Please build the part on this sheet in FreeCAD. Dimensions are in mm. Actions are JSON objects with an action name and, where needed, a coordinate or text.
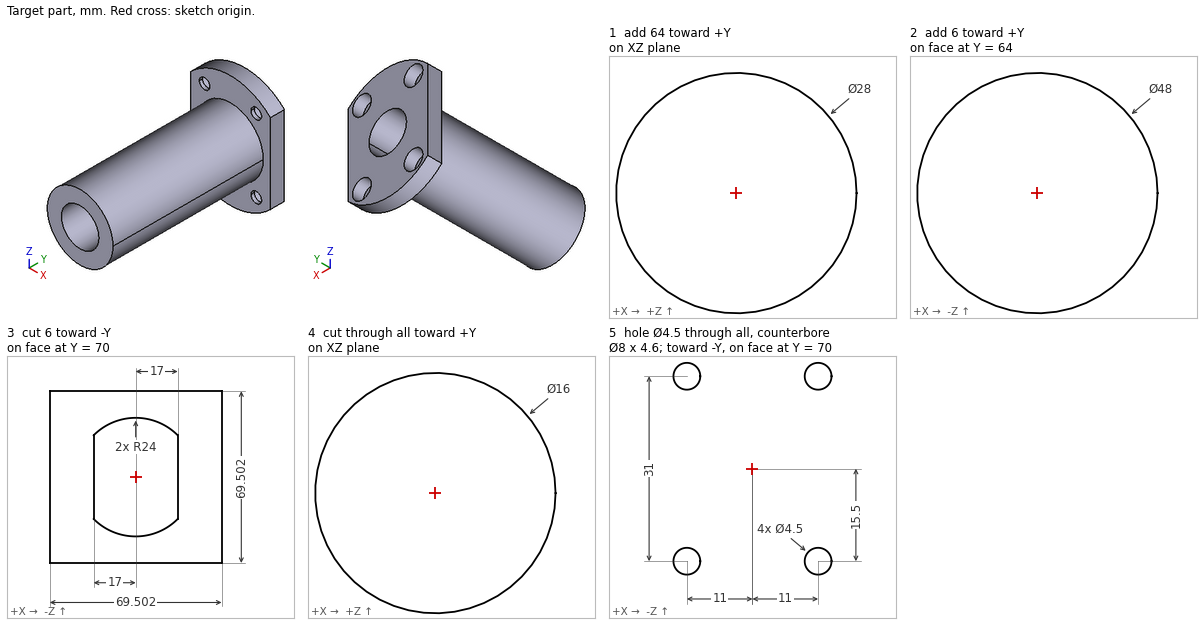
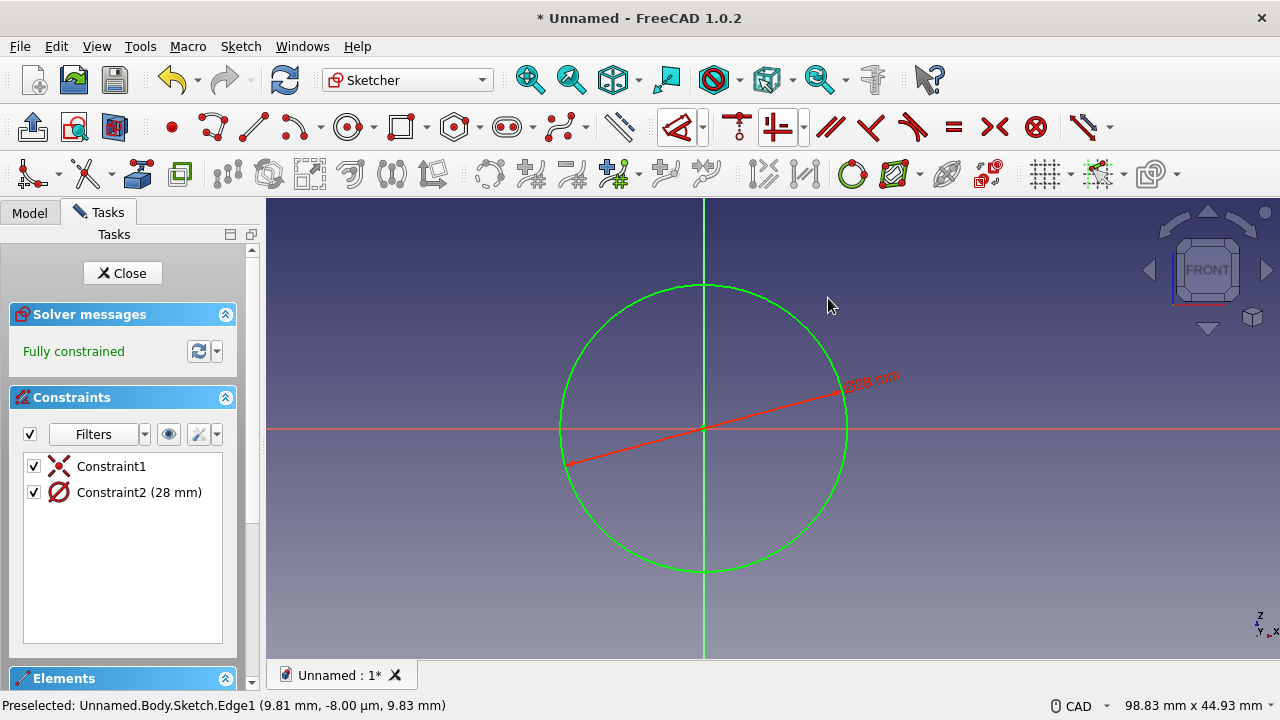
{"action": "left_click", "coordinate": [123, 273]}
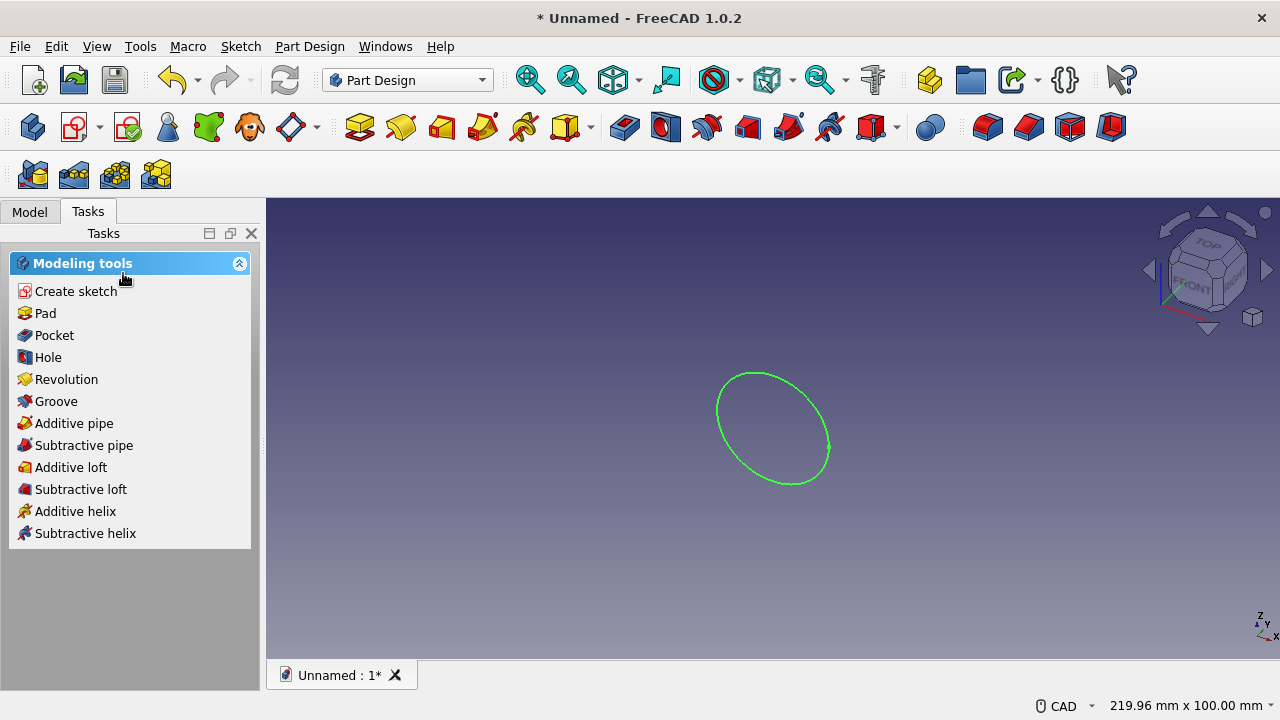
{"action": "left_click", "coordinate": [360, 128]}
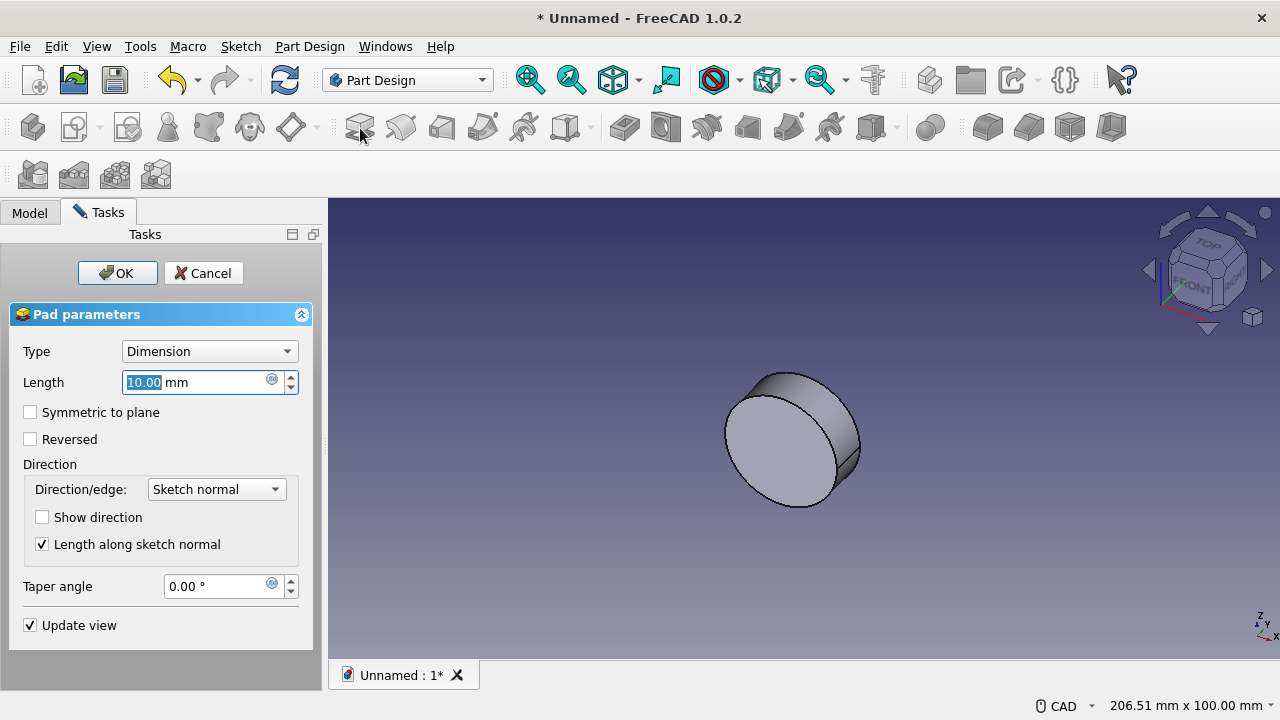
{"action": "type", "text": "64"}
{"action": "key", "text": "Tab"}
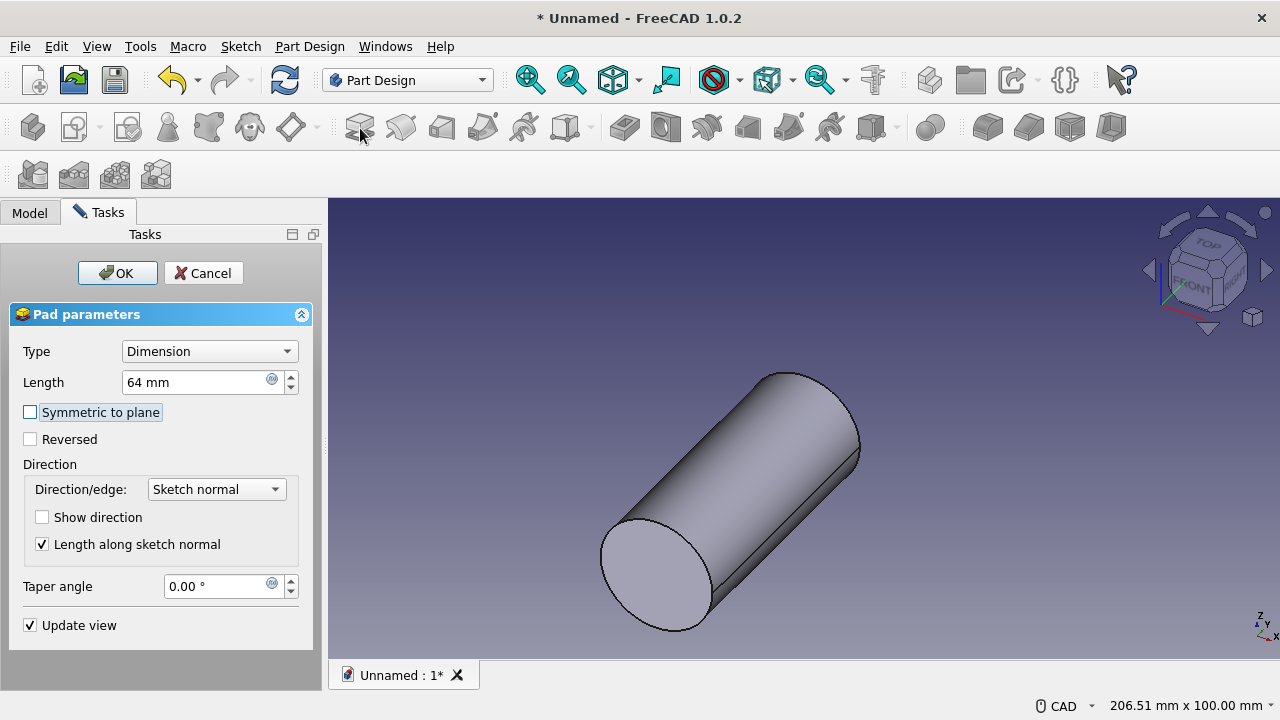
{"action": "left_click", "coordinate": [31, 439]}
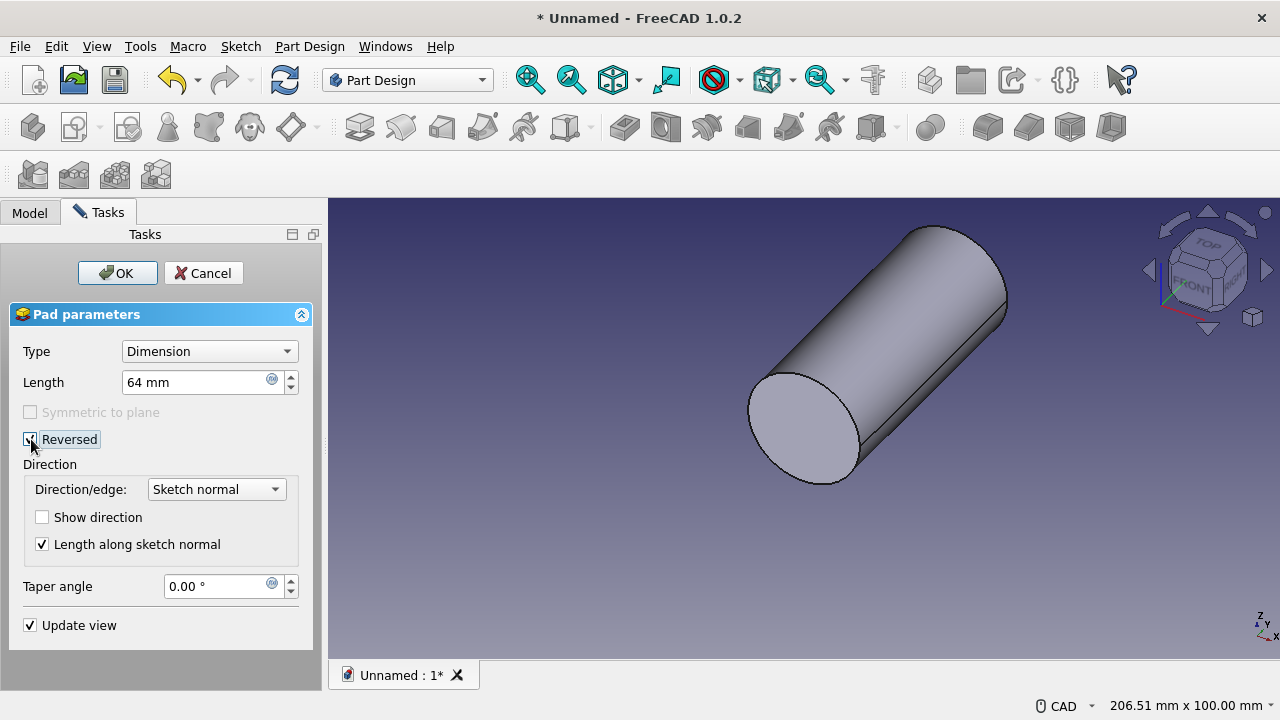
{"action": "left_click", "coordinate": [118, 273]}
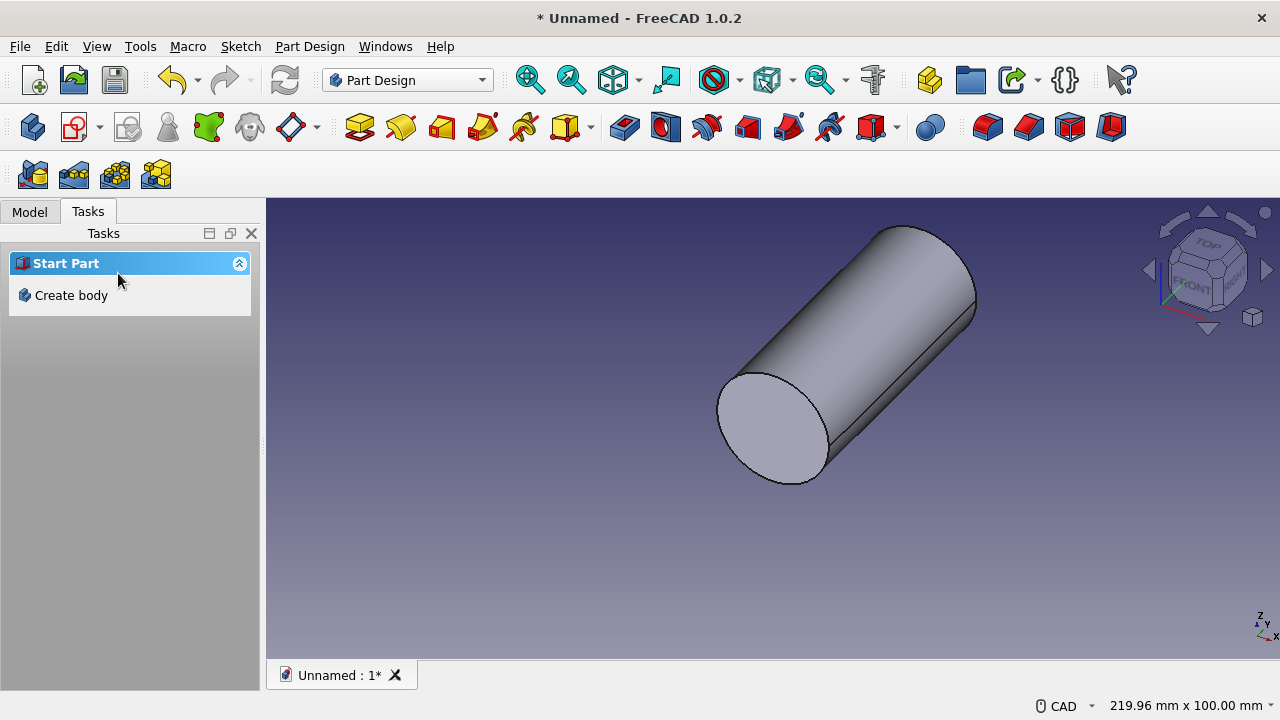
{"action": "key", "text": "4"}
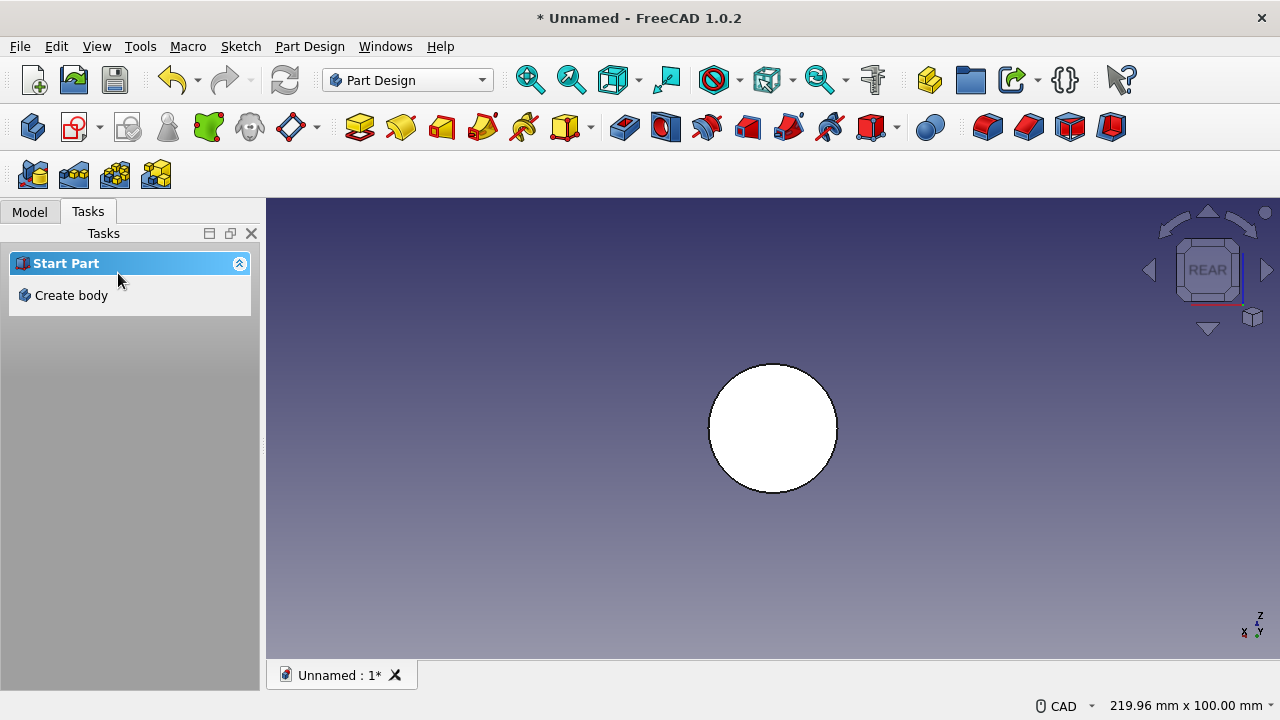
{"action": "left_click", "coordinate": [531, 80]}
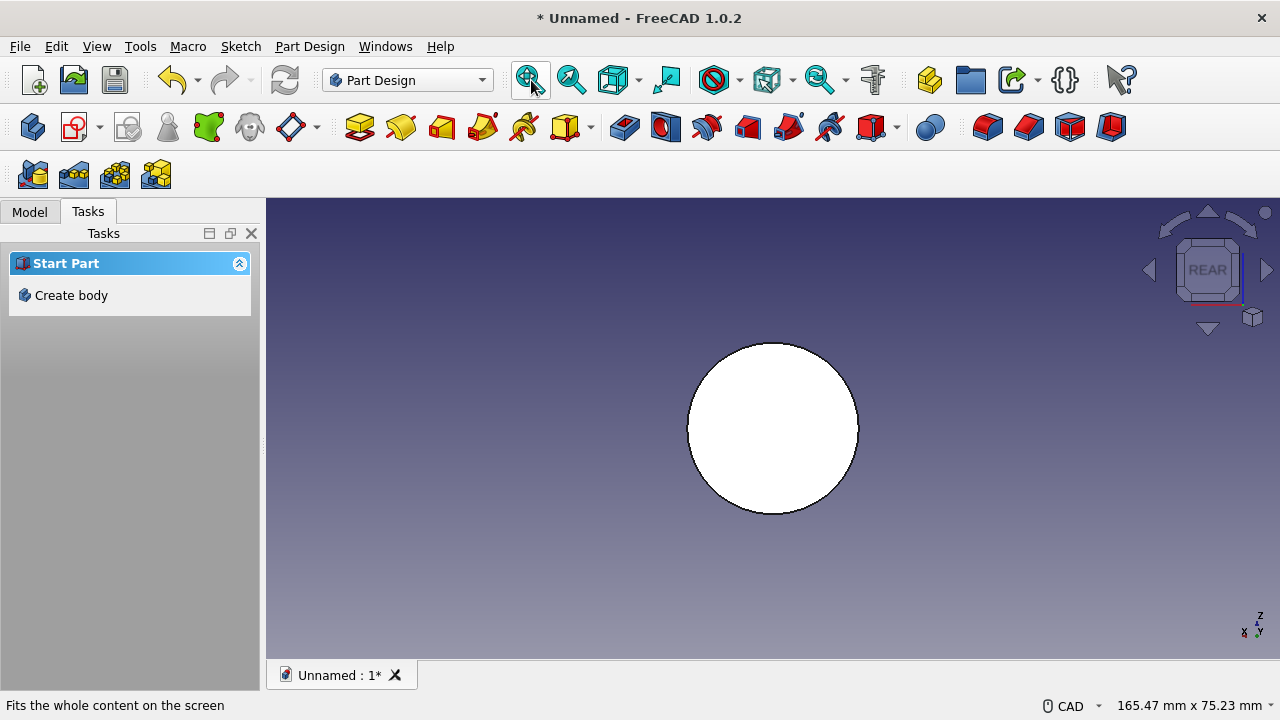
{"action": "left_click", "coordinate": [773, 428]}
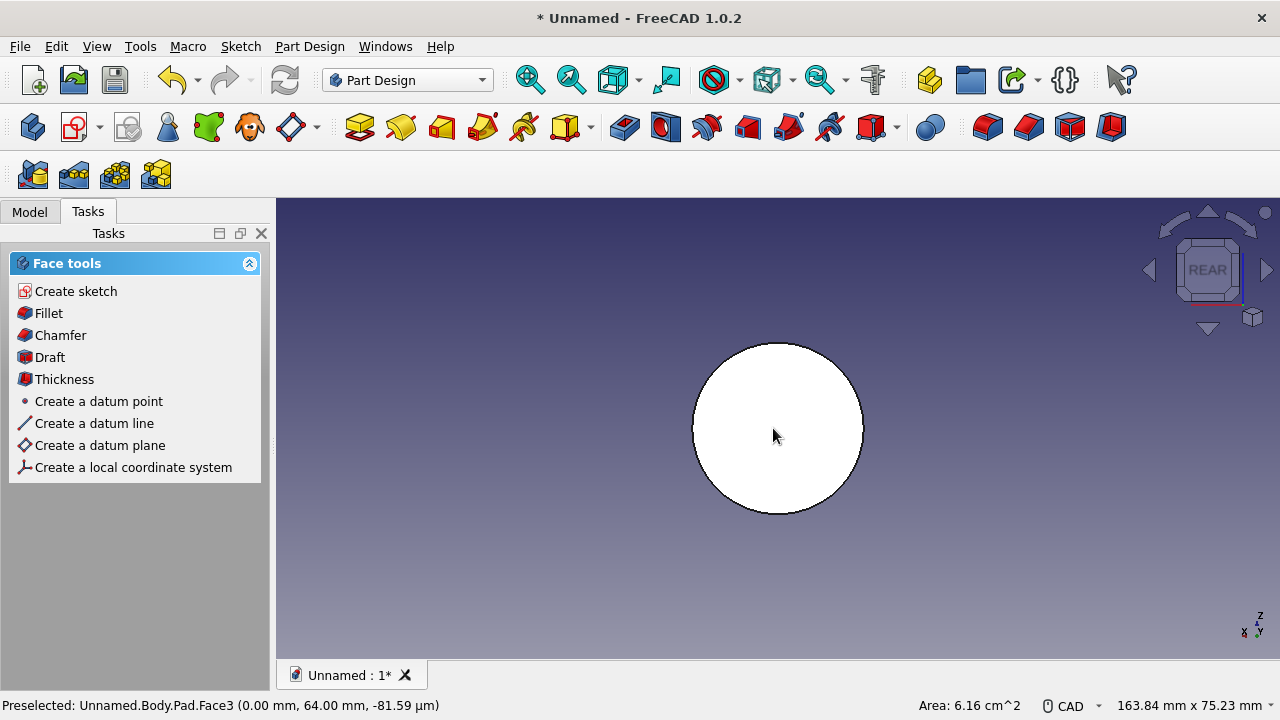
{"action": "left_click", "coordinate": [74, 128]}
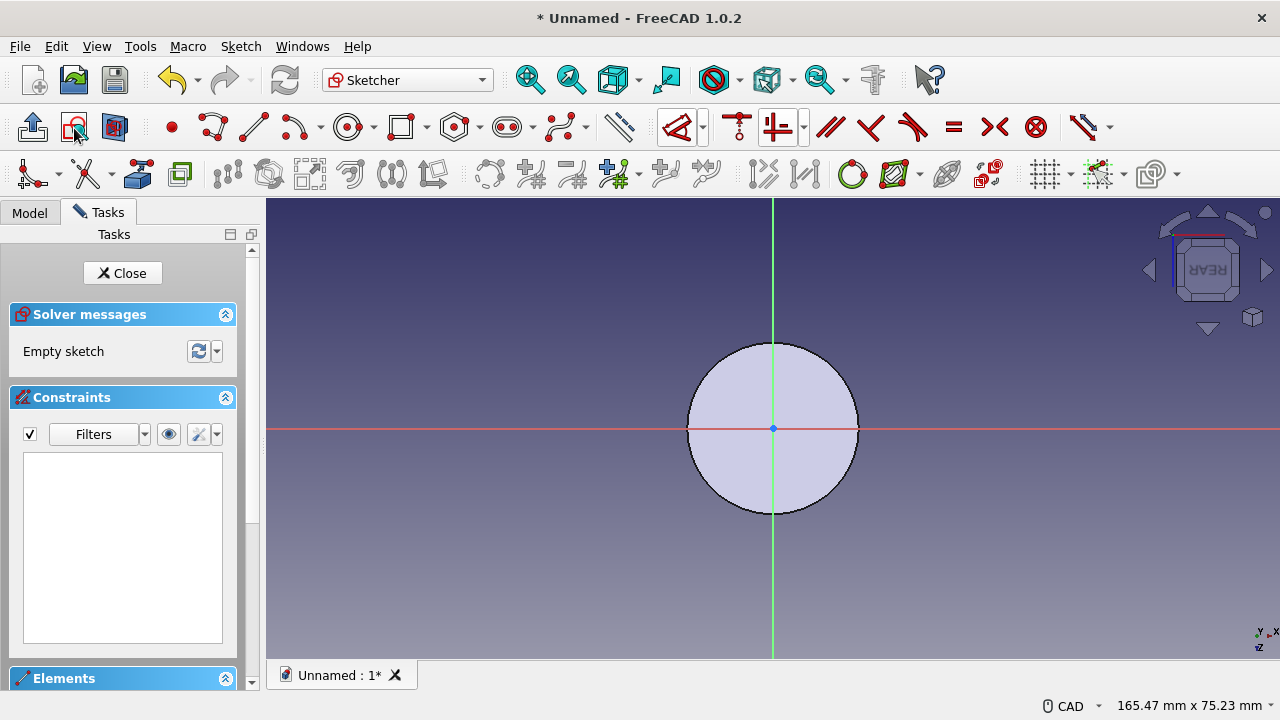
{"action": "left_click", "coordinate": [348, 128]}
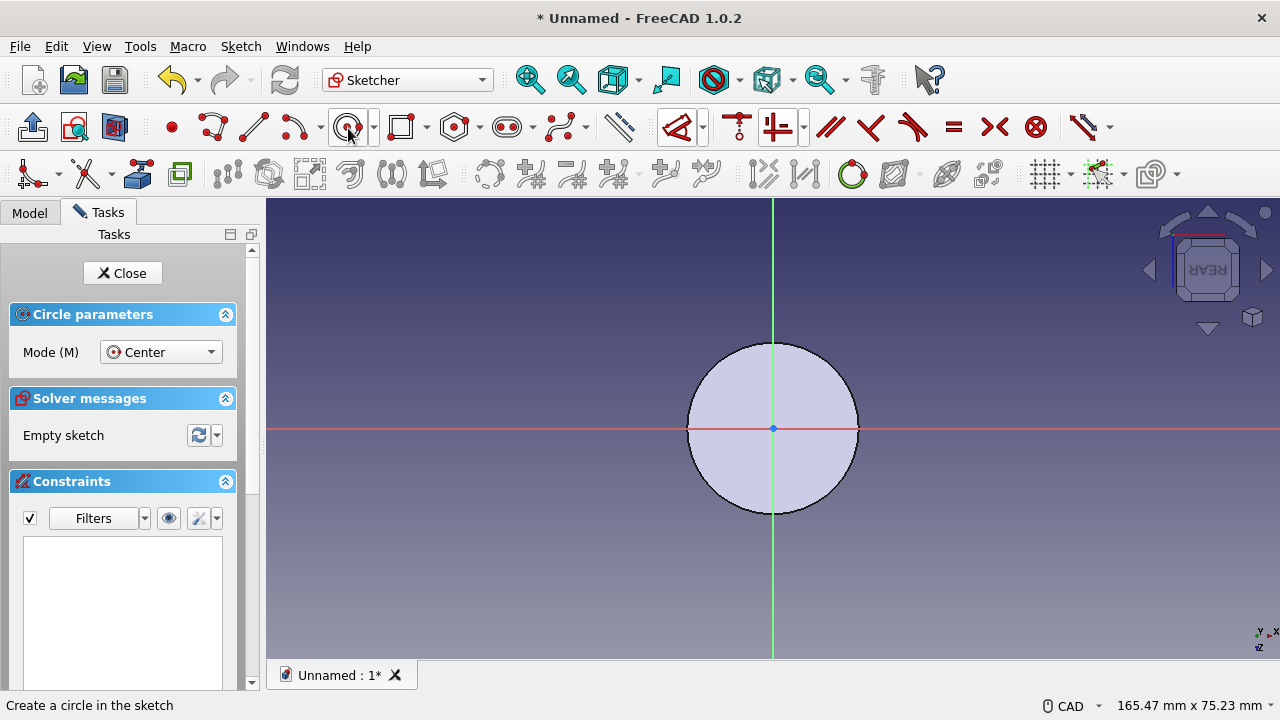
{"action": "left_click", "coordinate": [773, 428]}
{"action": "left_click", "coordinate": [877, 325]}
{"action": "key", "text": "Escape"}